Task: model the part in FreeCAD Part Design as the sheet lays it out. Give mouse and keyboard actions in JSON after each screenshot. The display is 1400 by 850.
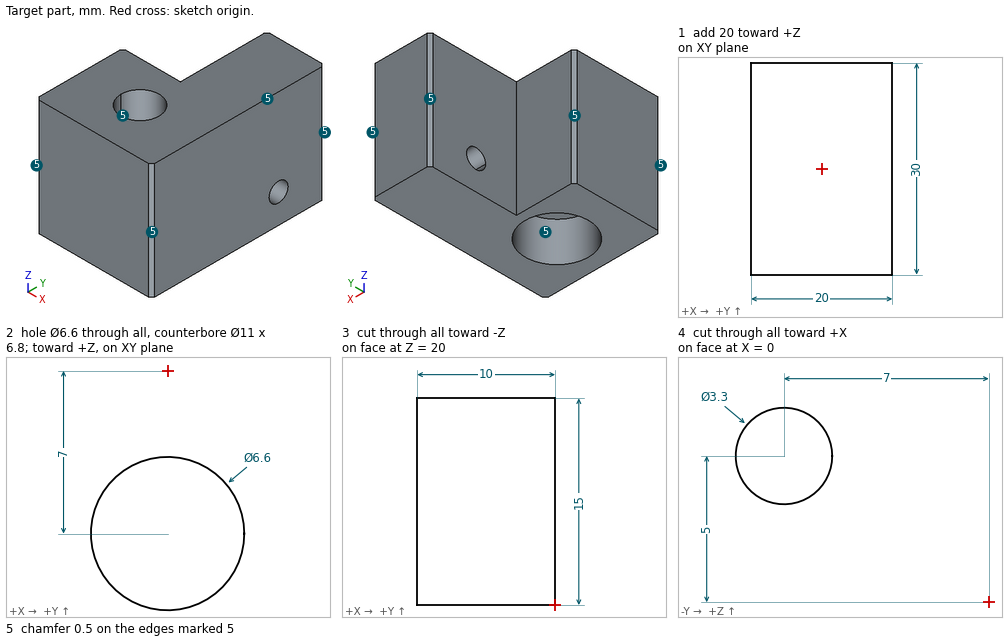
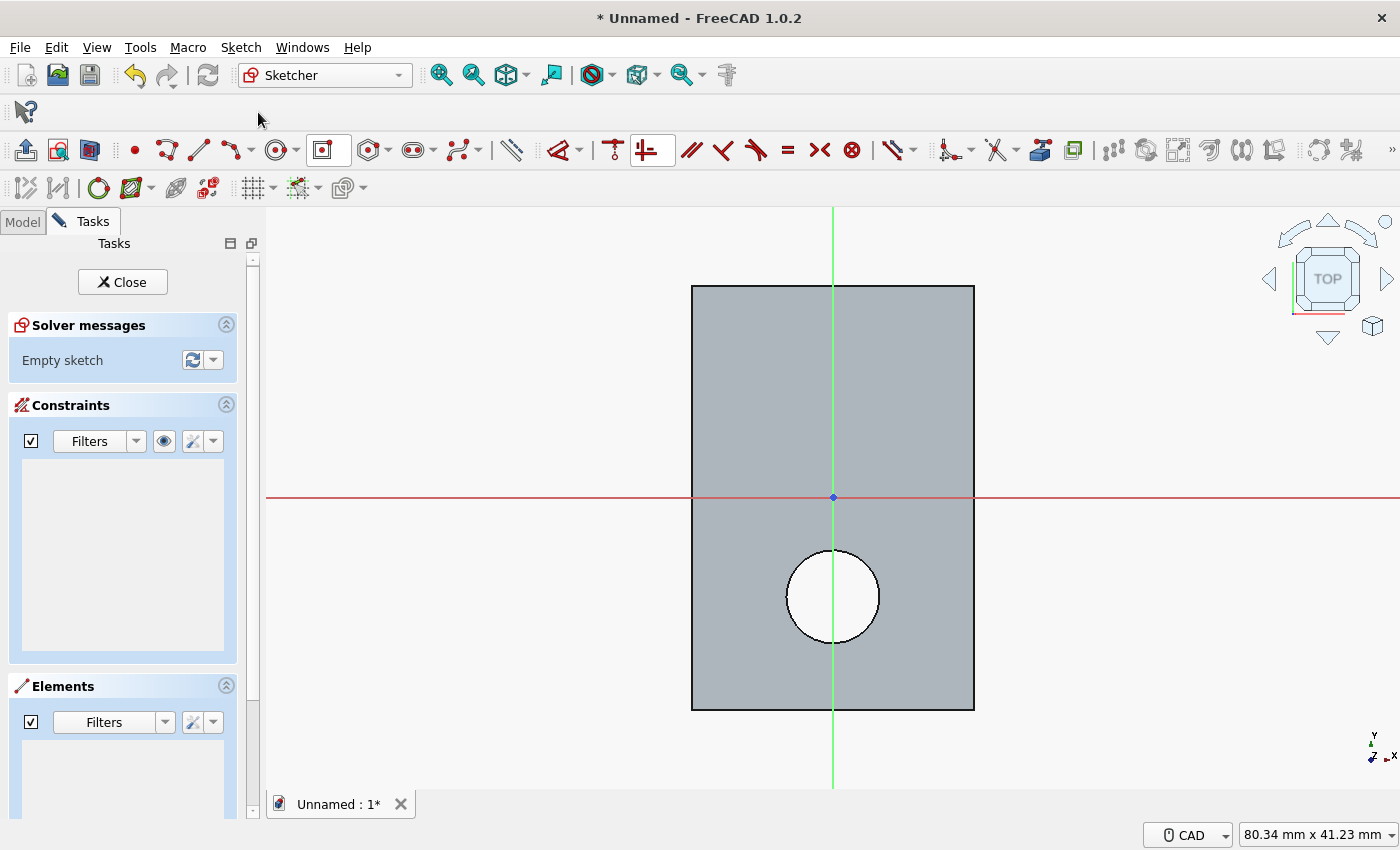
{"action": "scroll", "coordinate": [760, 263], "scroll_direction": "up", "scroll_amount": 3}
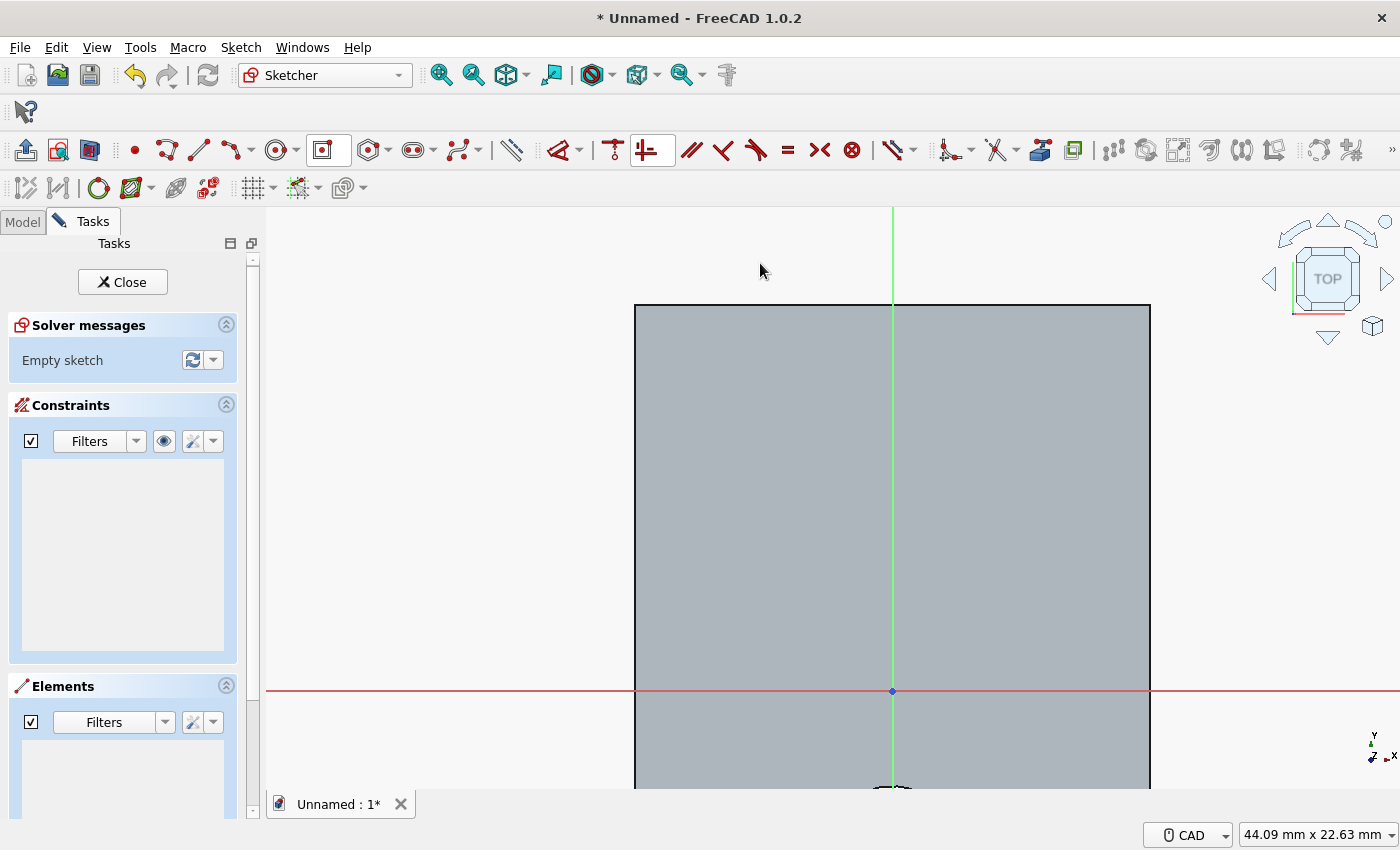
{"action": "key", "text": "g r"}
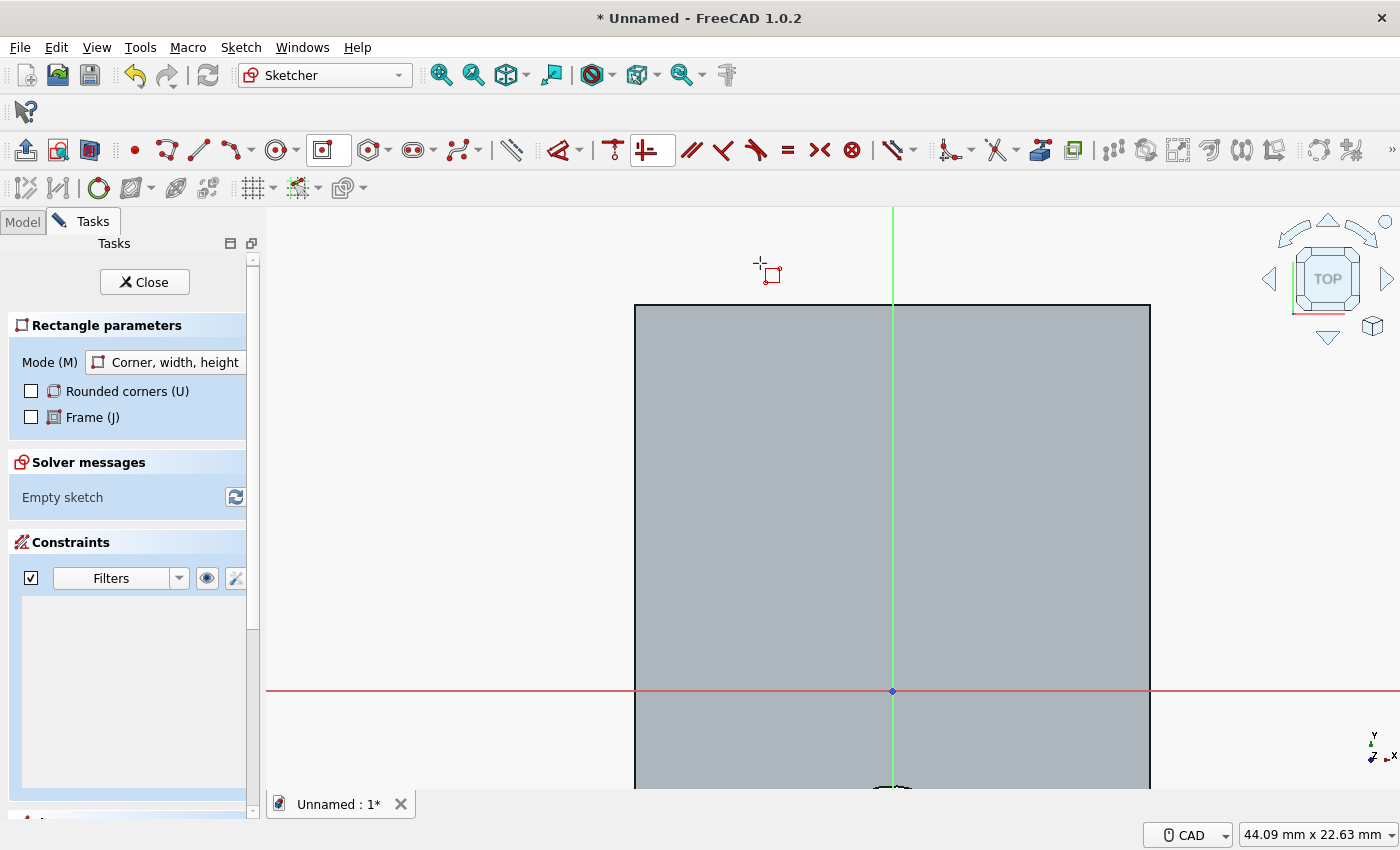
{"action": "left_click", "coordinate": [893, 691]}
{"action": "left_click", "coordinate": [635, 305]}
{"action": "key", "text": "Escape"}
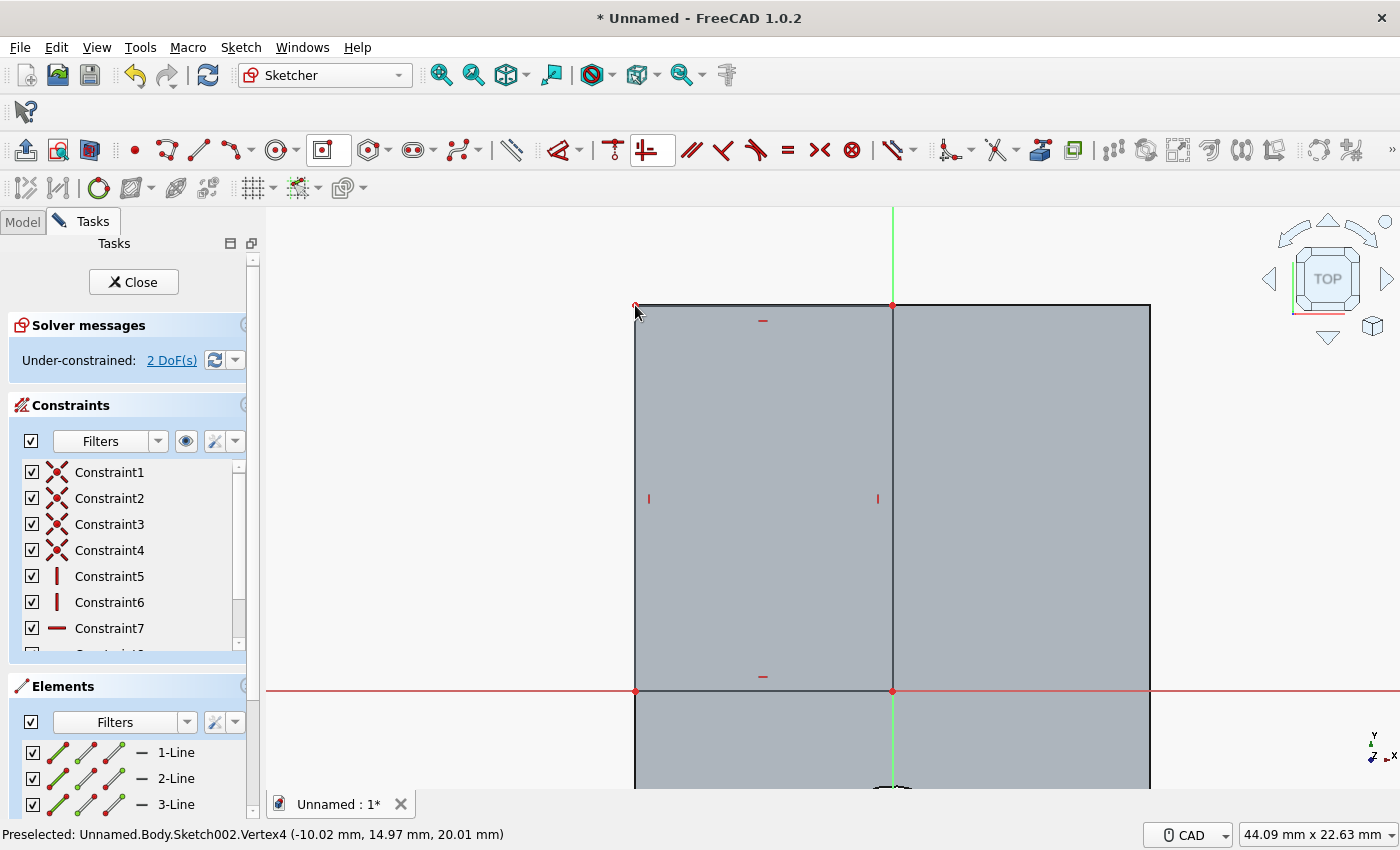
{"action": "left_click", "coordinate": [558, 150]}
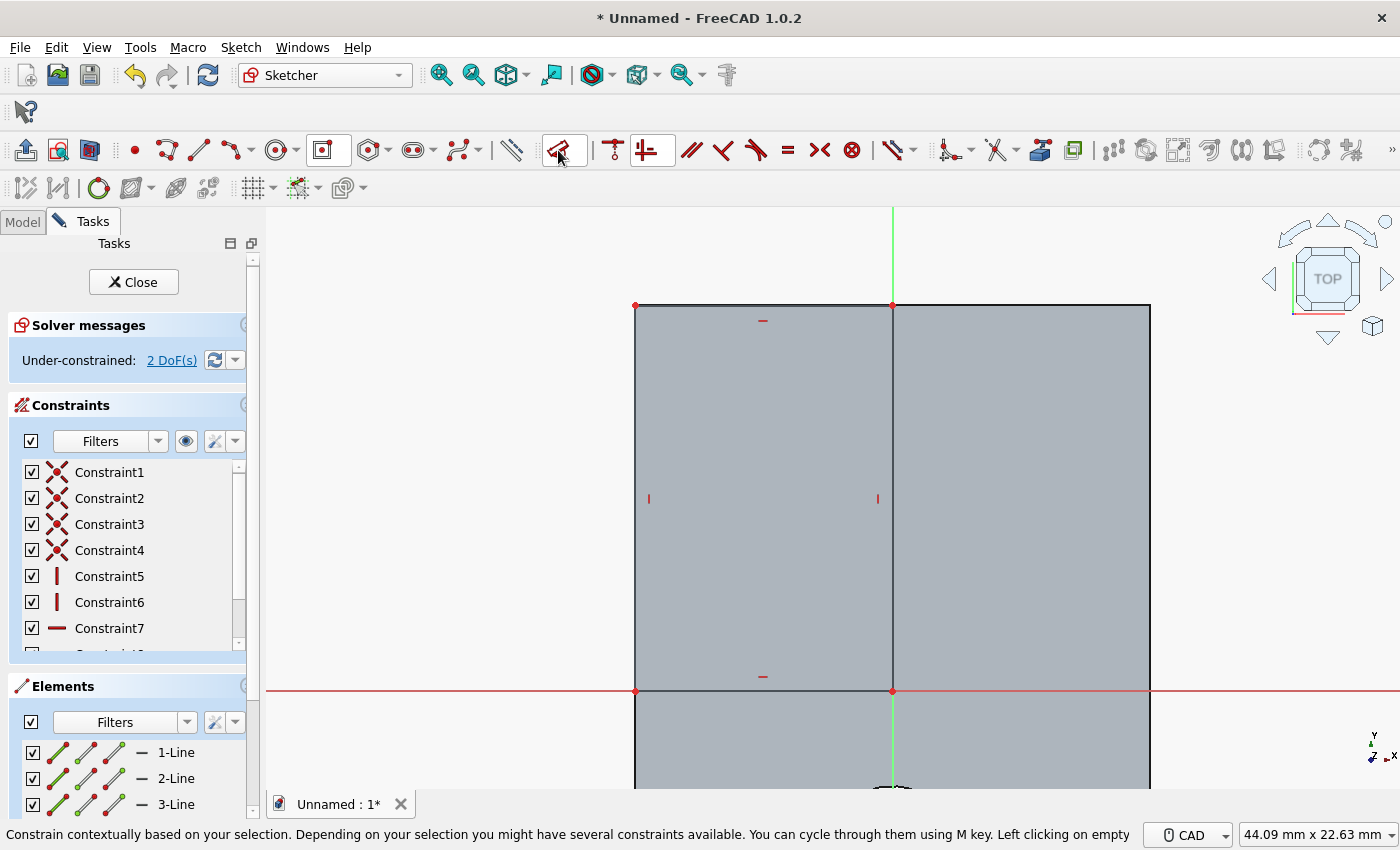
{"action": "left_click", "coordinate": [893, 576]}
{"action": "left_click", "coordinate": [927, 499]}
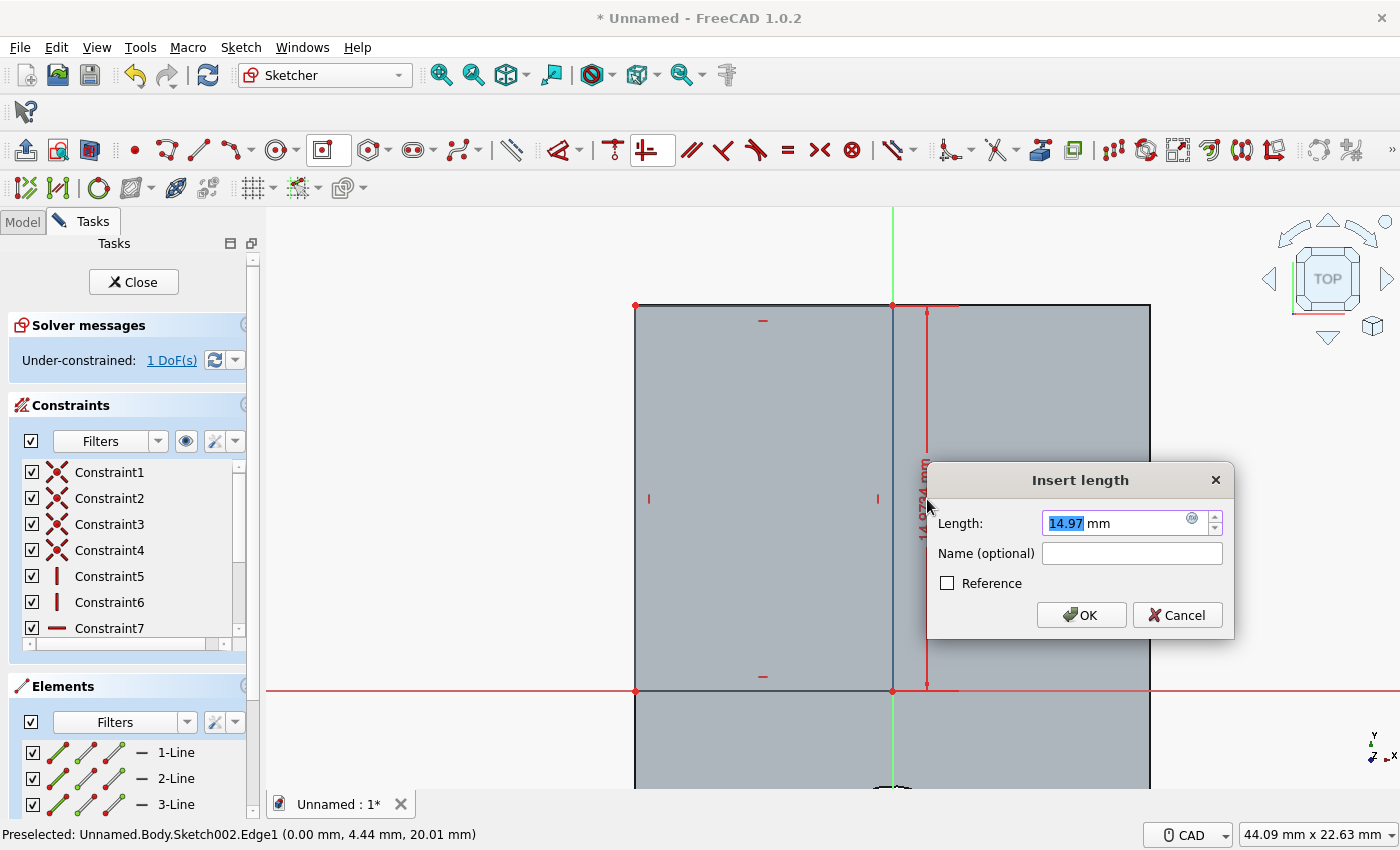
{"action": "type", "text": "15"}
{"action": "key", "text": "Return"}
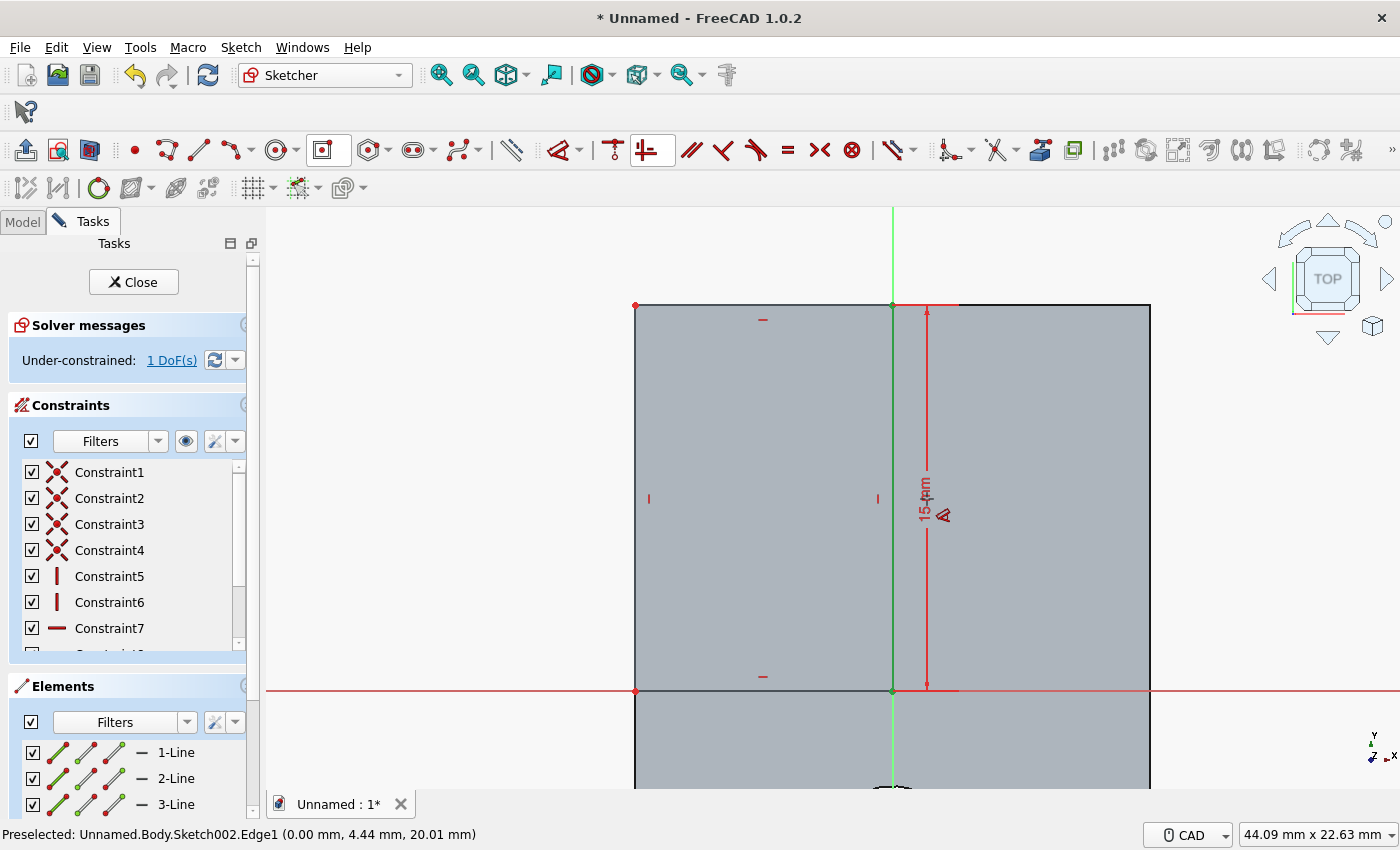
{"action": "left_click", "coordinate": [815, 305]}
{"action": "left_click", "coordinate": [764, 271]}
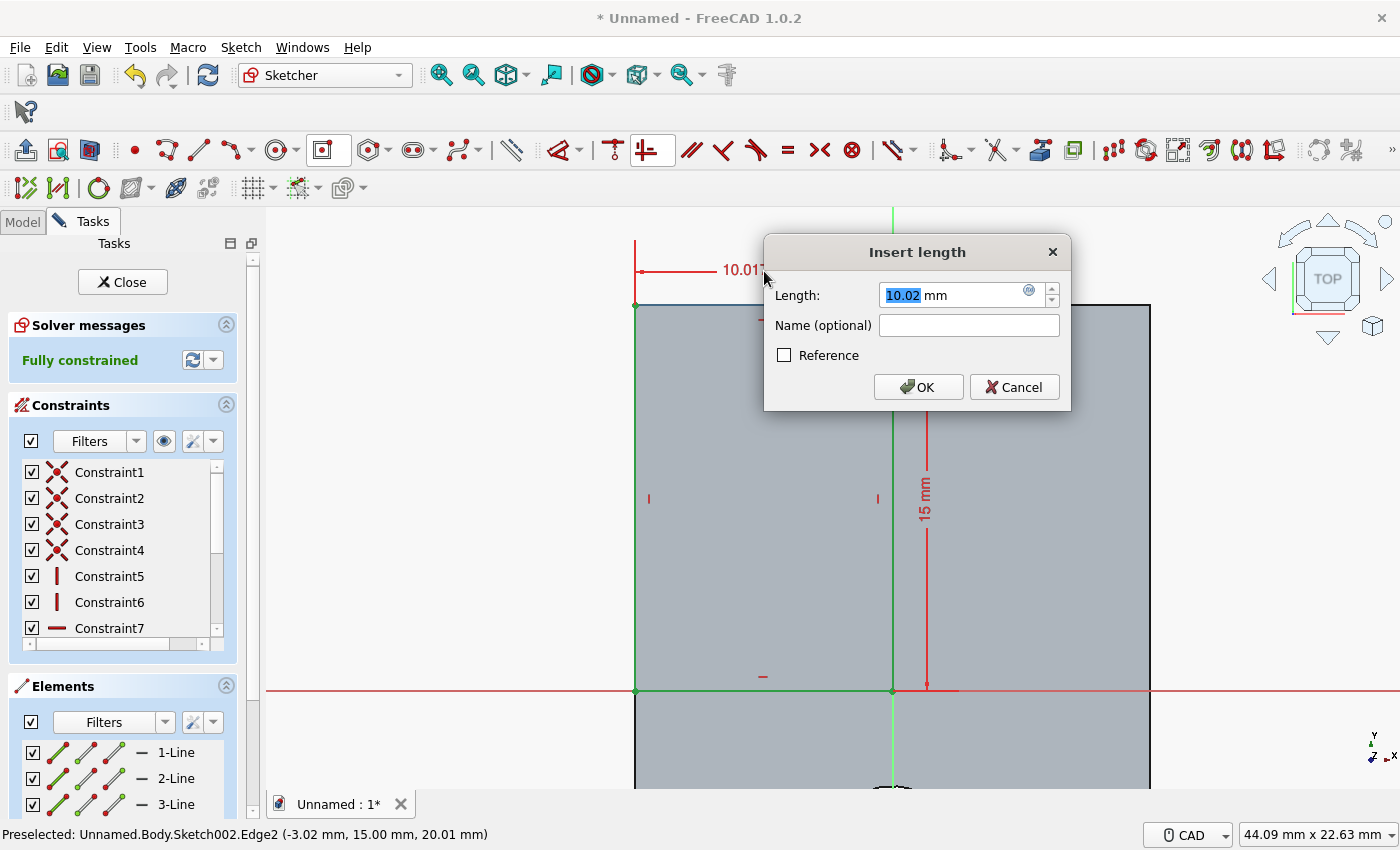
{"action": "type", "text": "10"}
{"action": "key", "text": "Return"}
{"action": "key", "text": "Escape"}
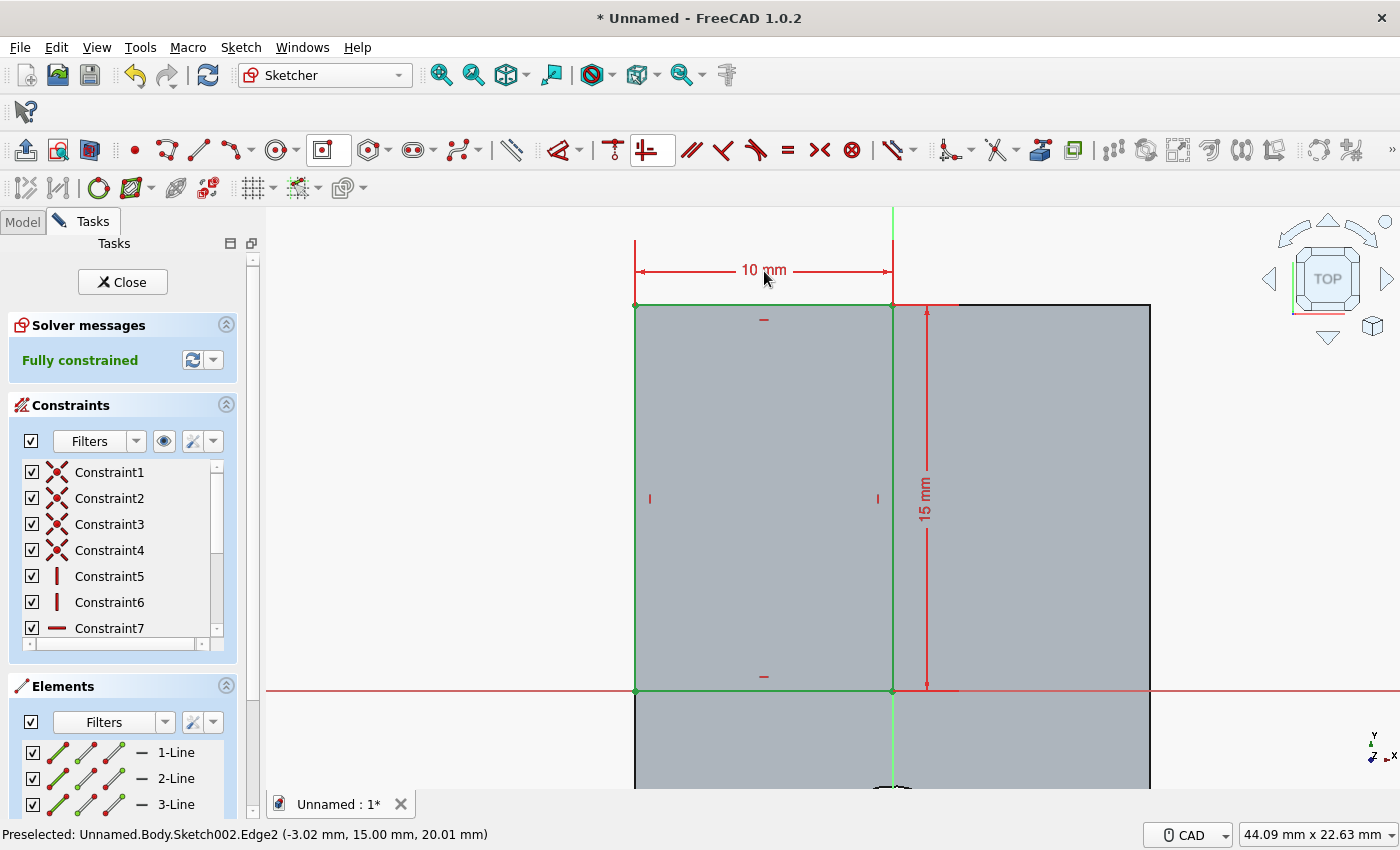
{"action": "left_click", "coordinate": [123, 282]}